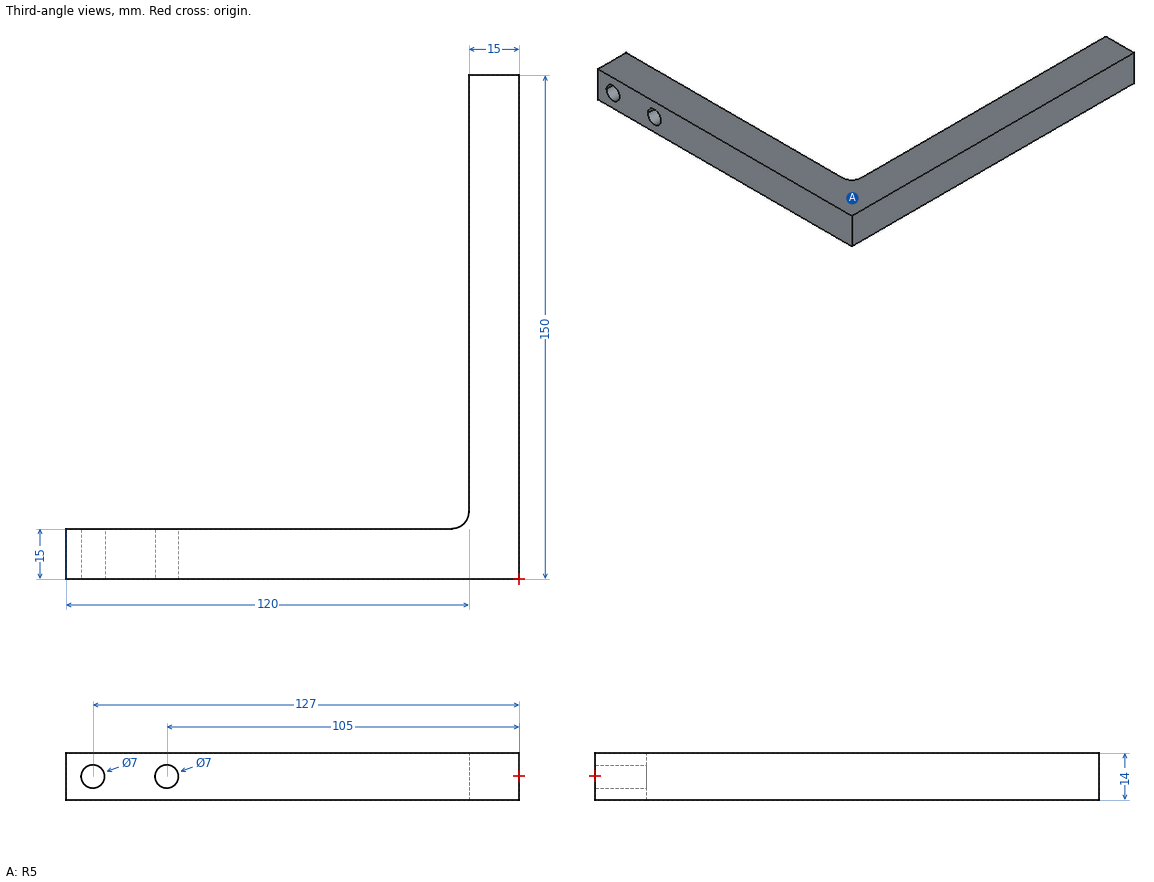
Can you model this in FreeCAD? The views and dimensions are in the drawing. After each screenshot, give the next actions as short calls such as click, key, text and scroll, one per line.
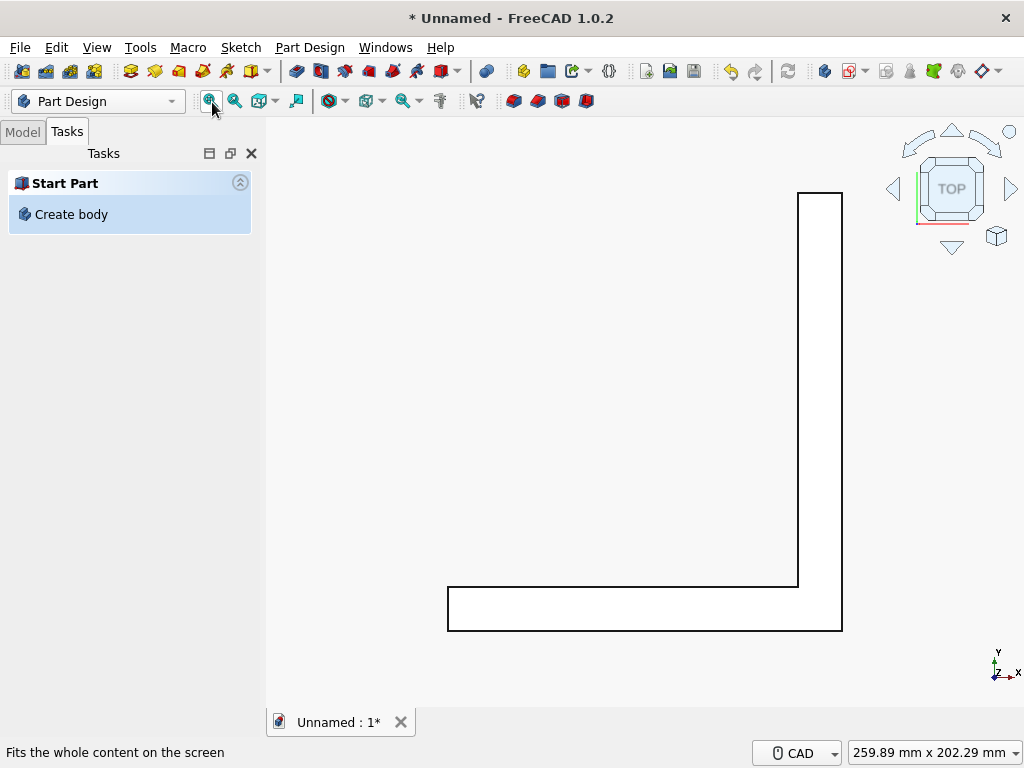
key(1)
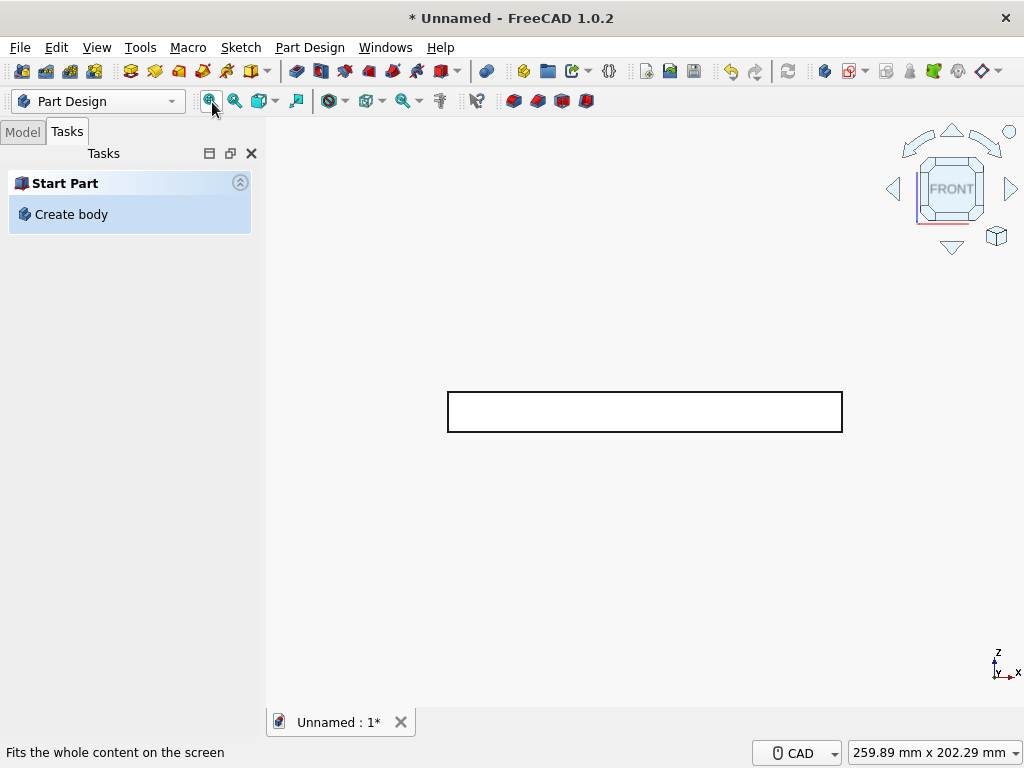
key(3)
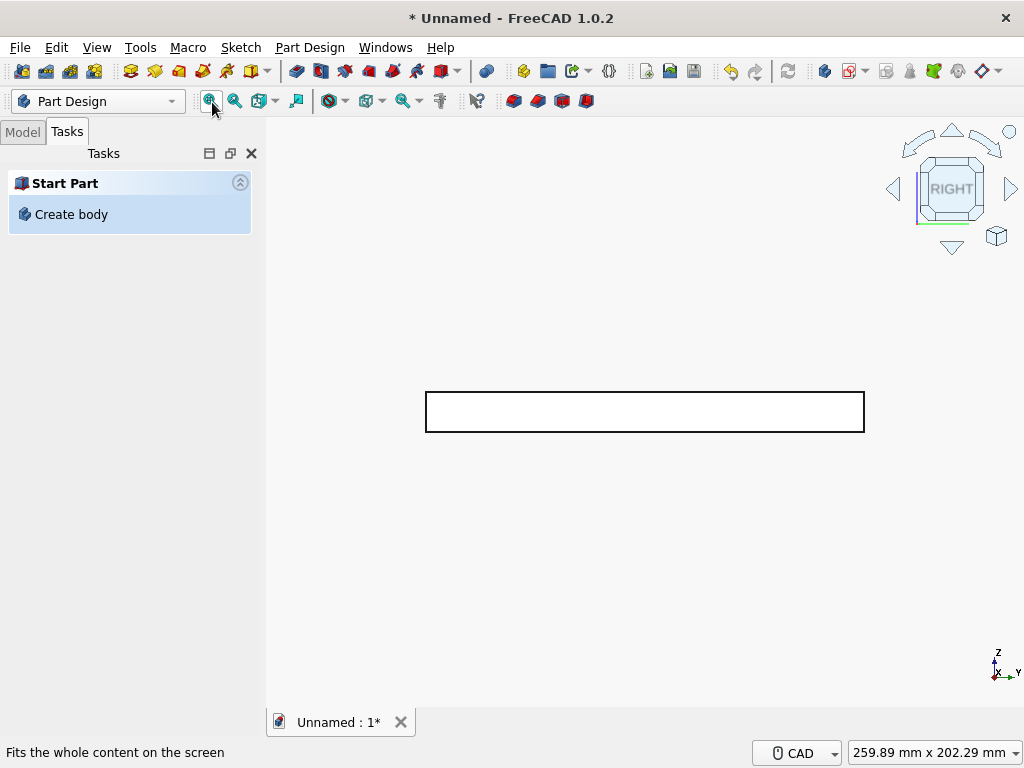
key(5)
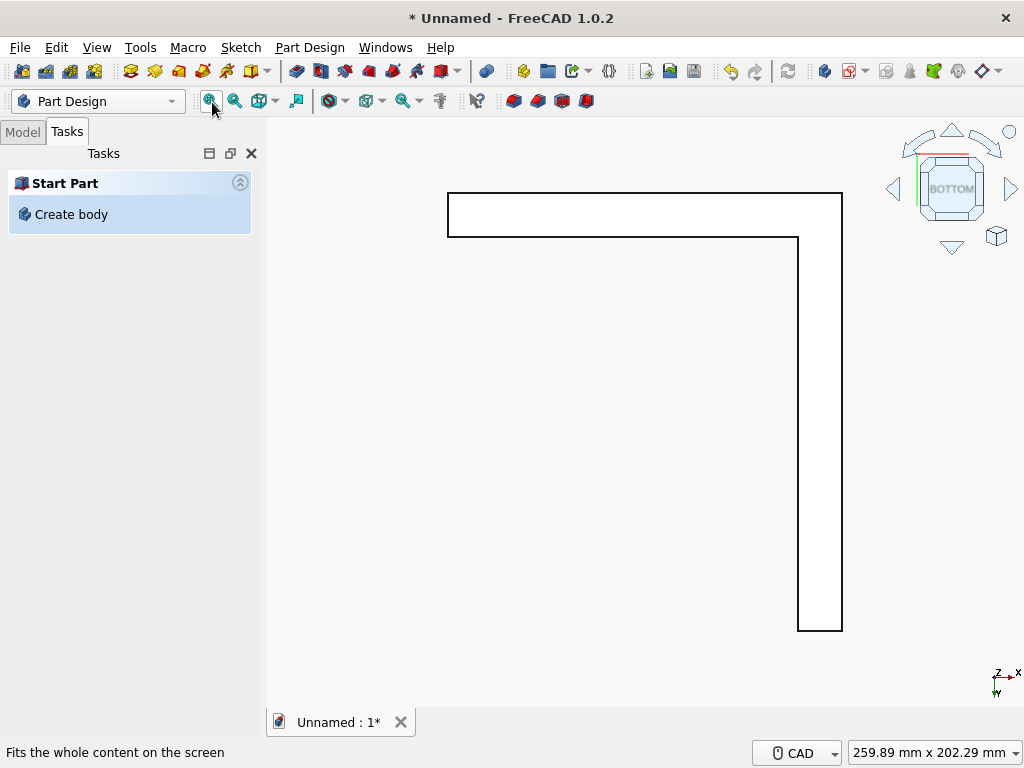
key(4)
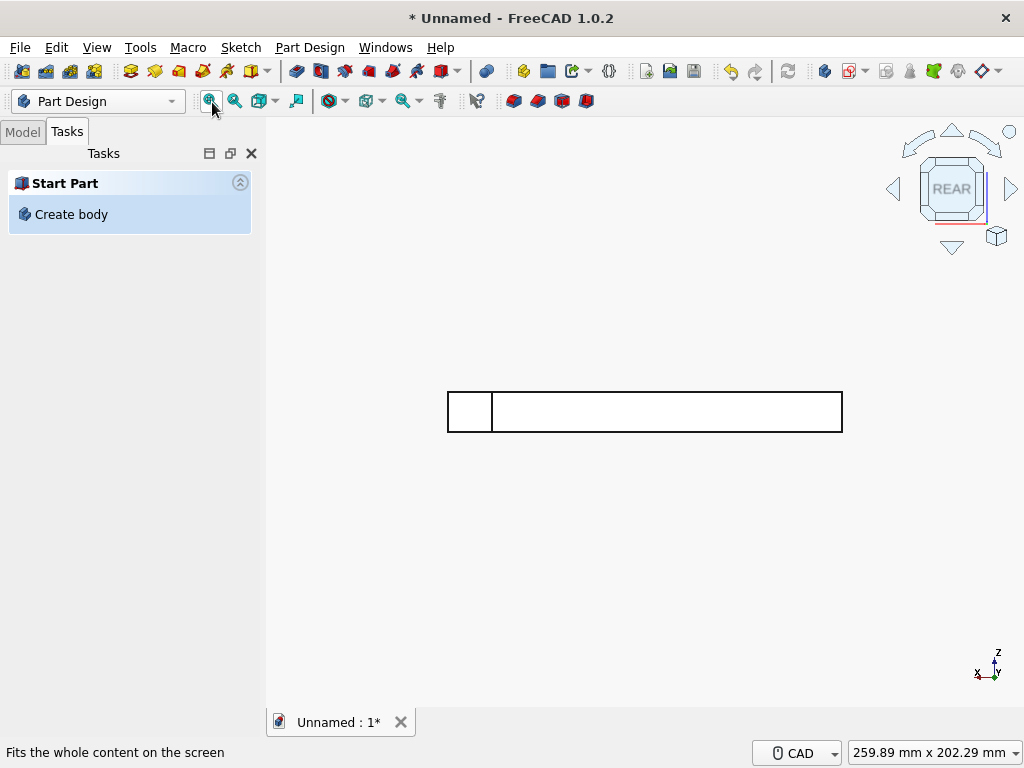
key(6)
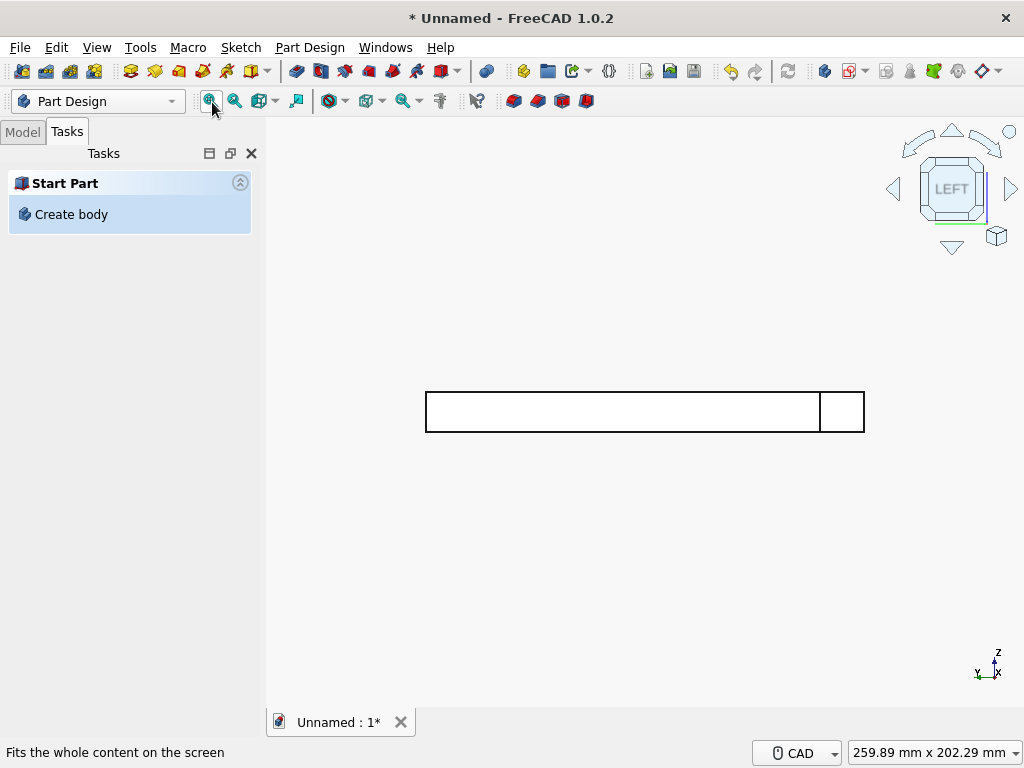
key(v)
key(3)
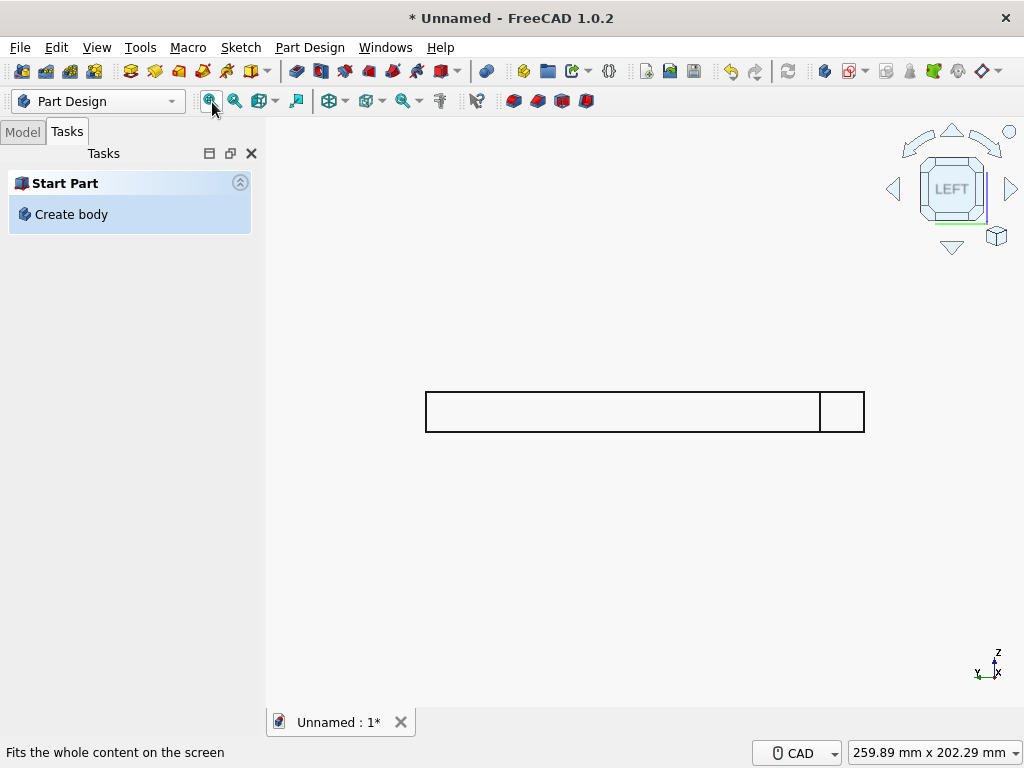
key(0)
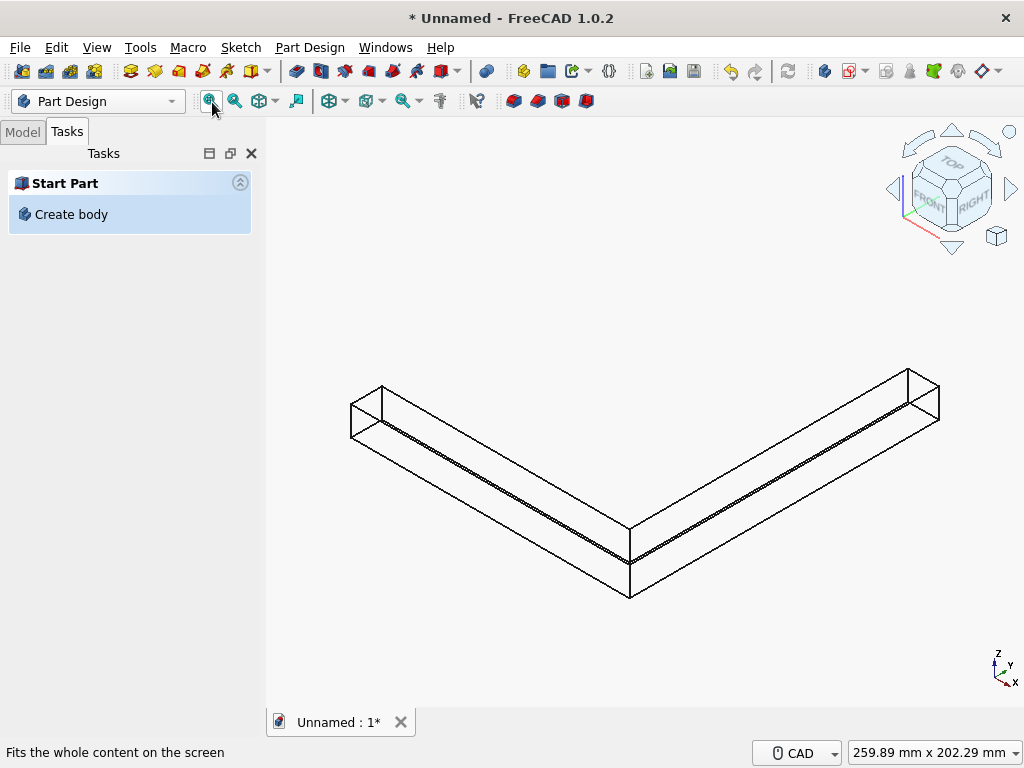
click(630, 545)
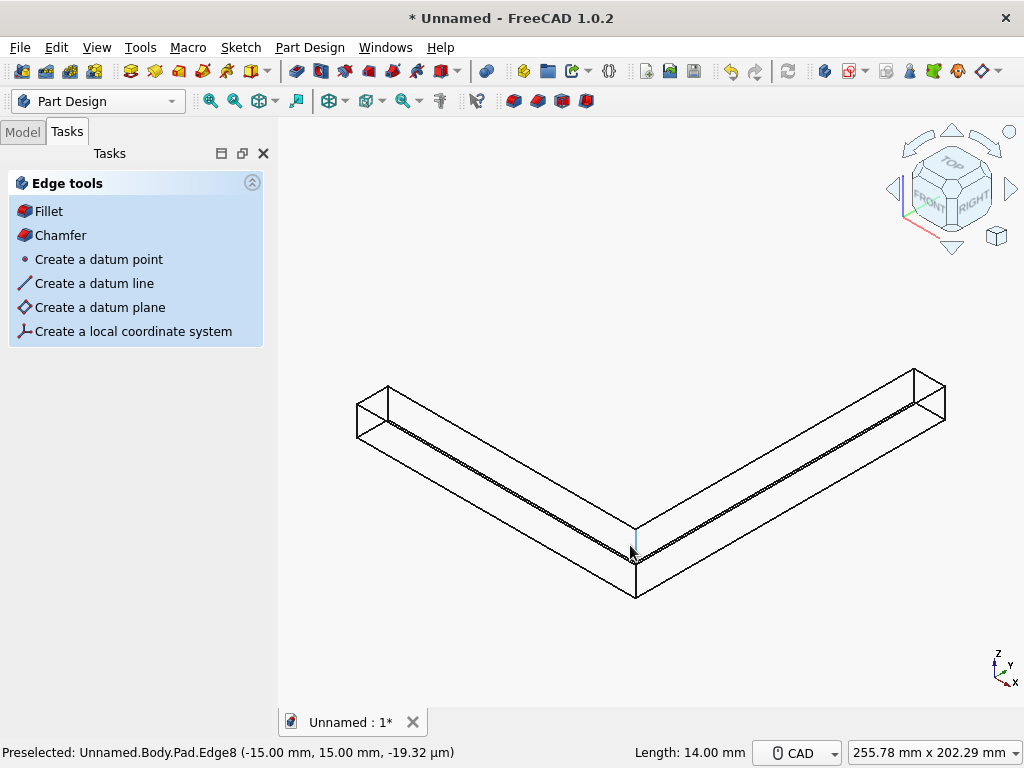
key(v)
key(1)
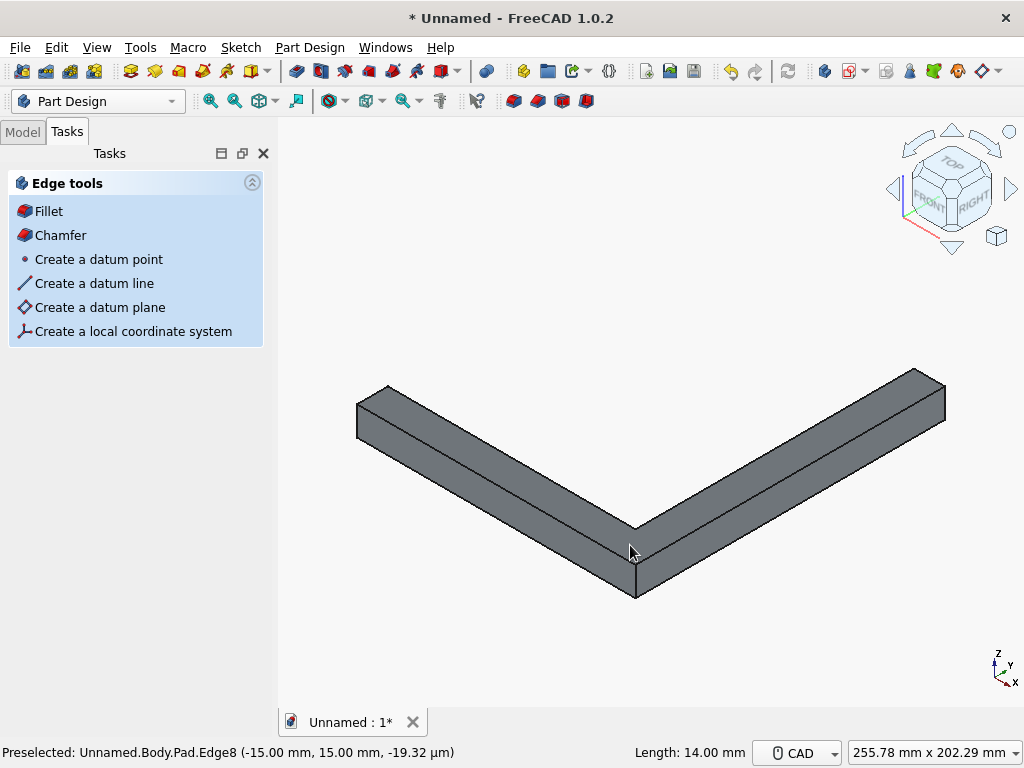
click(514, 102)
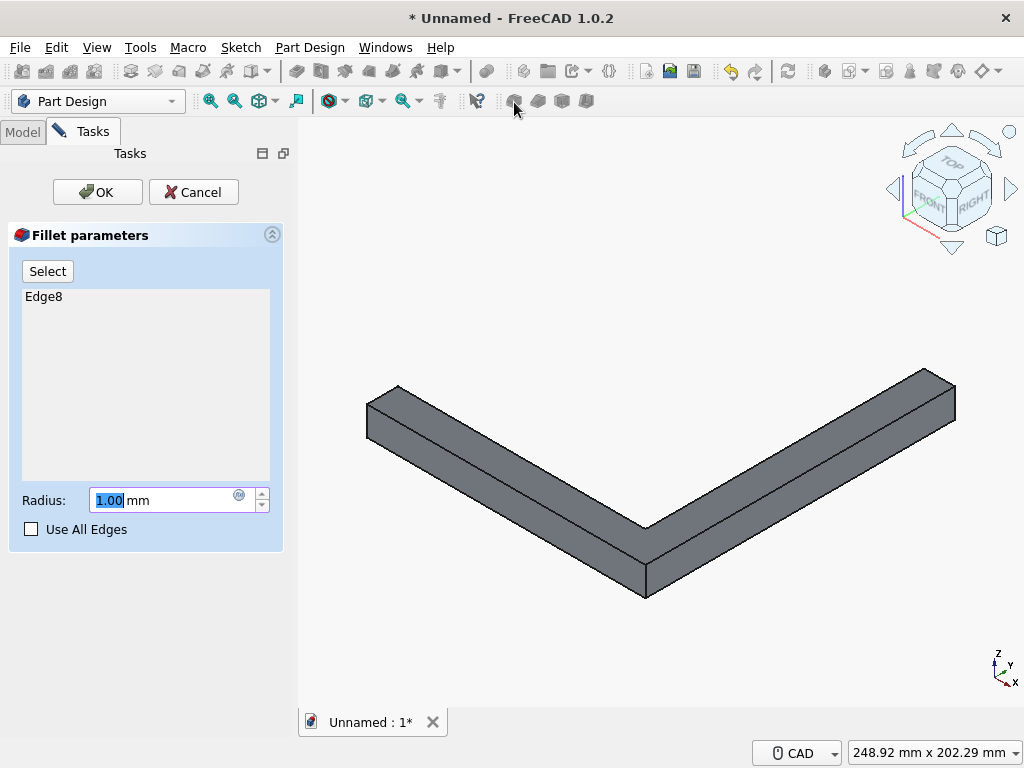
text(5)
key(Tab)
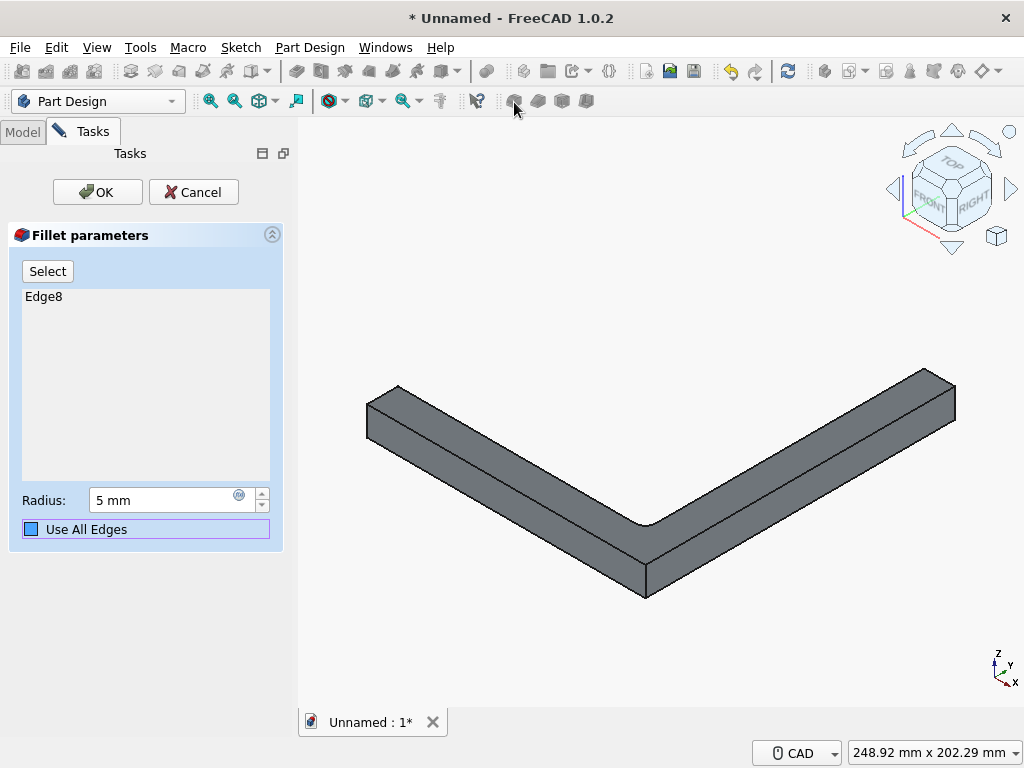
click(98, 192)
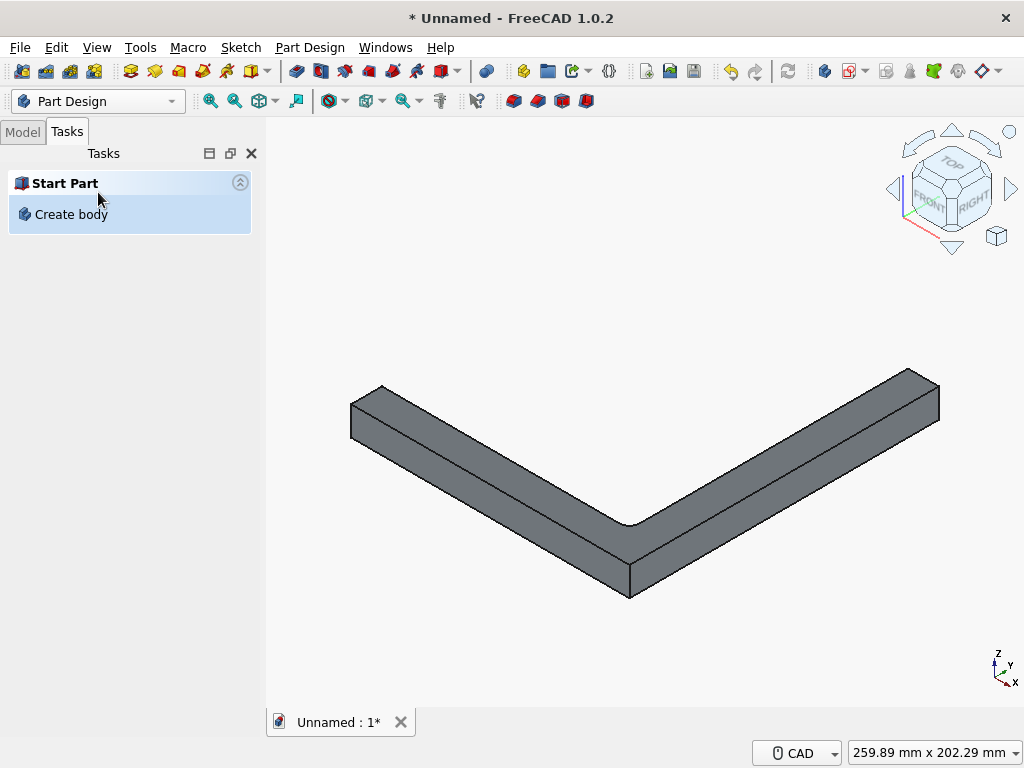
key(4)